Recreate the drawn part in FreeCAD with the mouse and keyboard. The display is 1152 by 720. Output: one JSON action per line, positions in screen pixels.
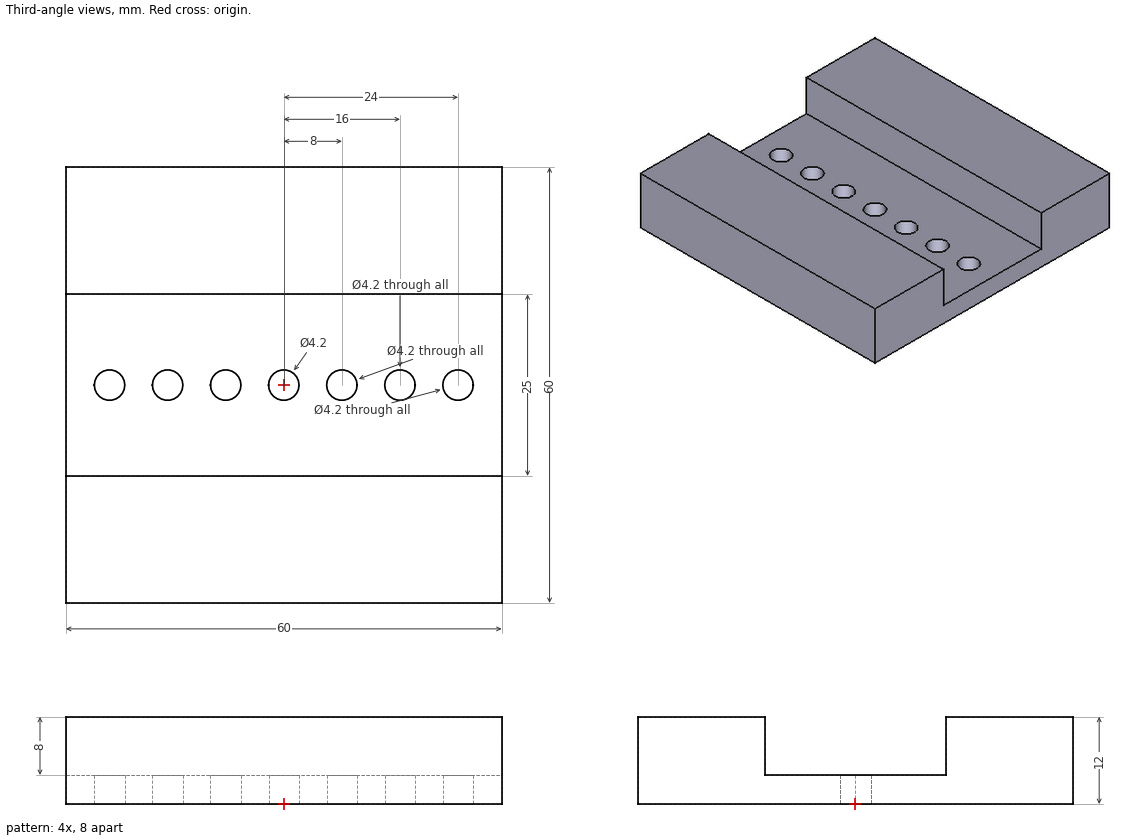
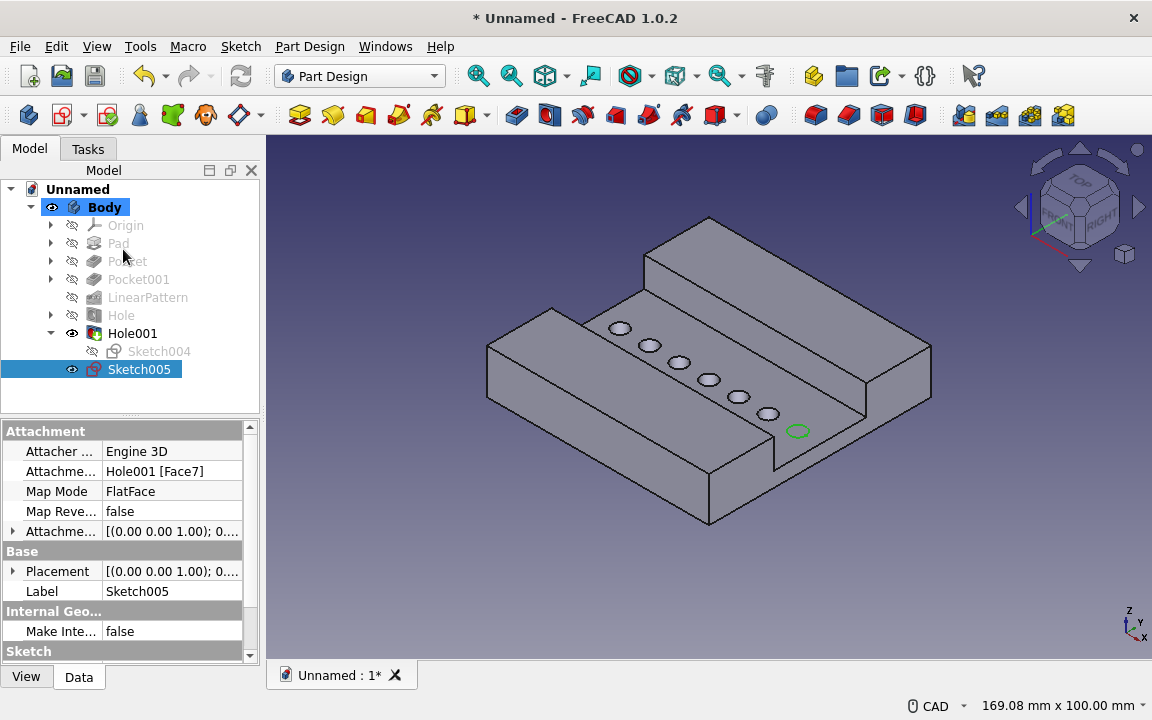
{"action": "left_click", "coordinate": [550, 116]}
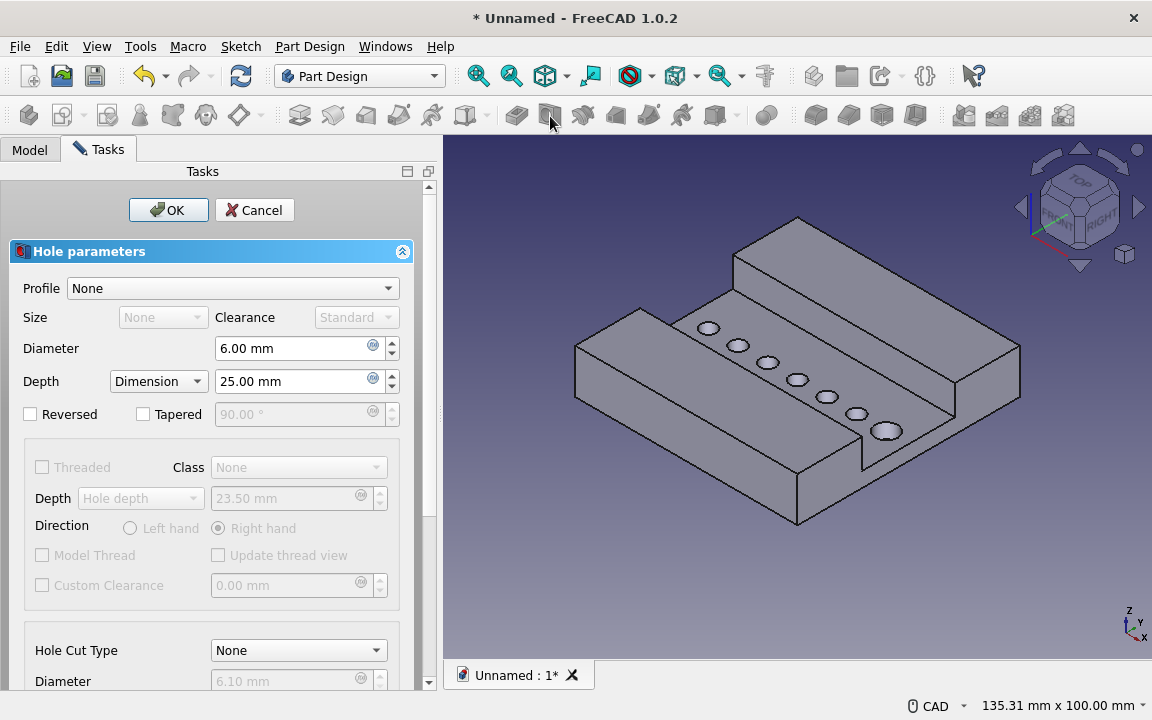
{"action": "triple_click", "coordinate": [300, 348]}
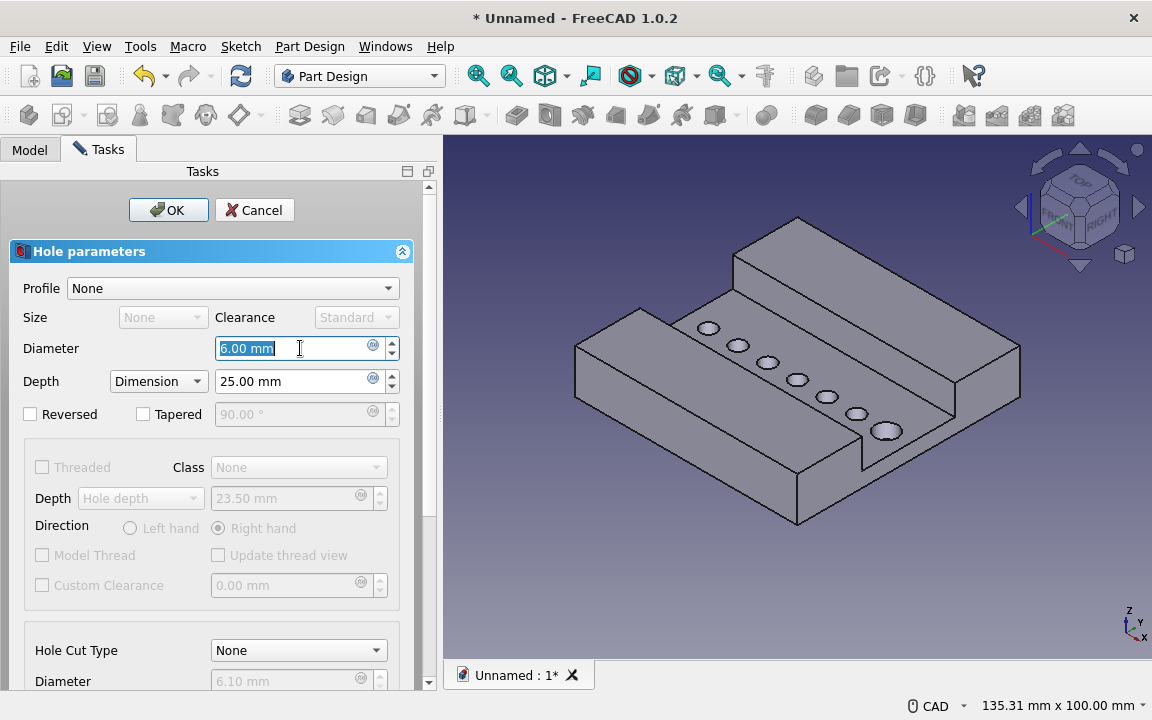
{"action": "type", "text": "4.2"}
{"action": "key", "text": "Tab"}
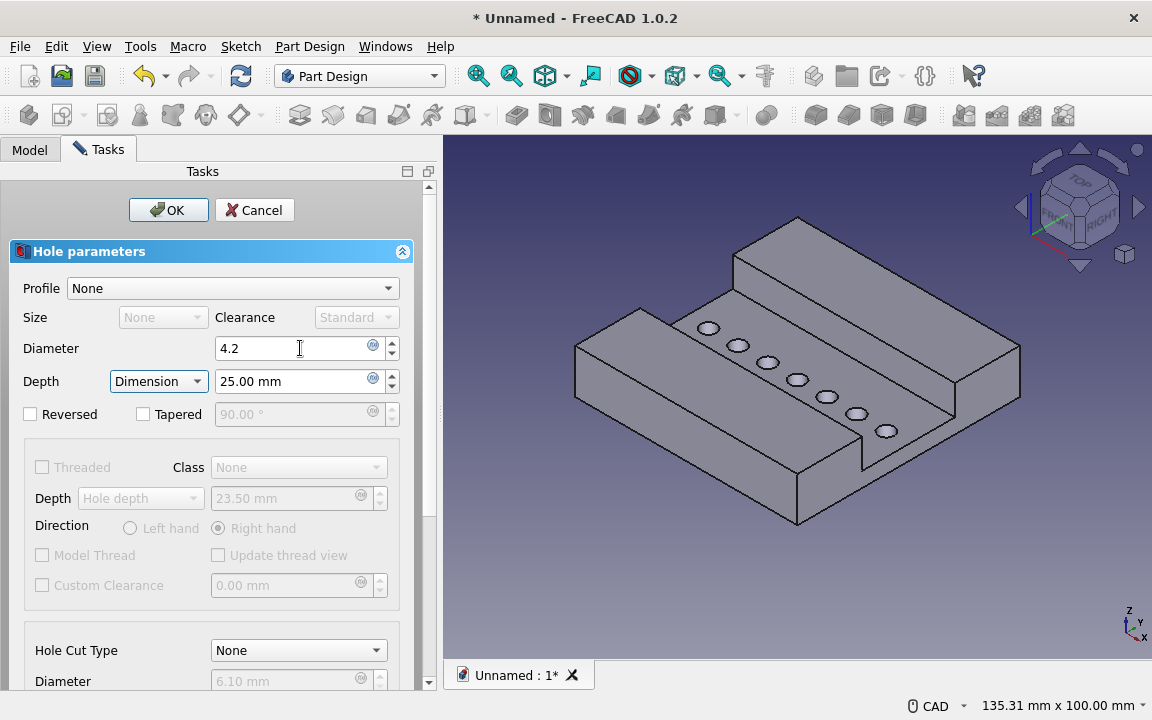
{"action": "left_click", "coordinate": [160, 382]}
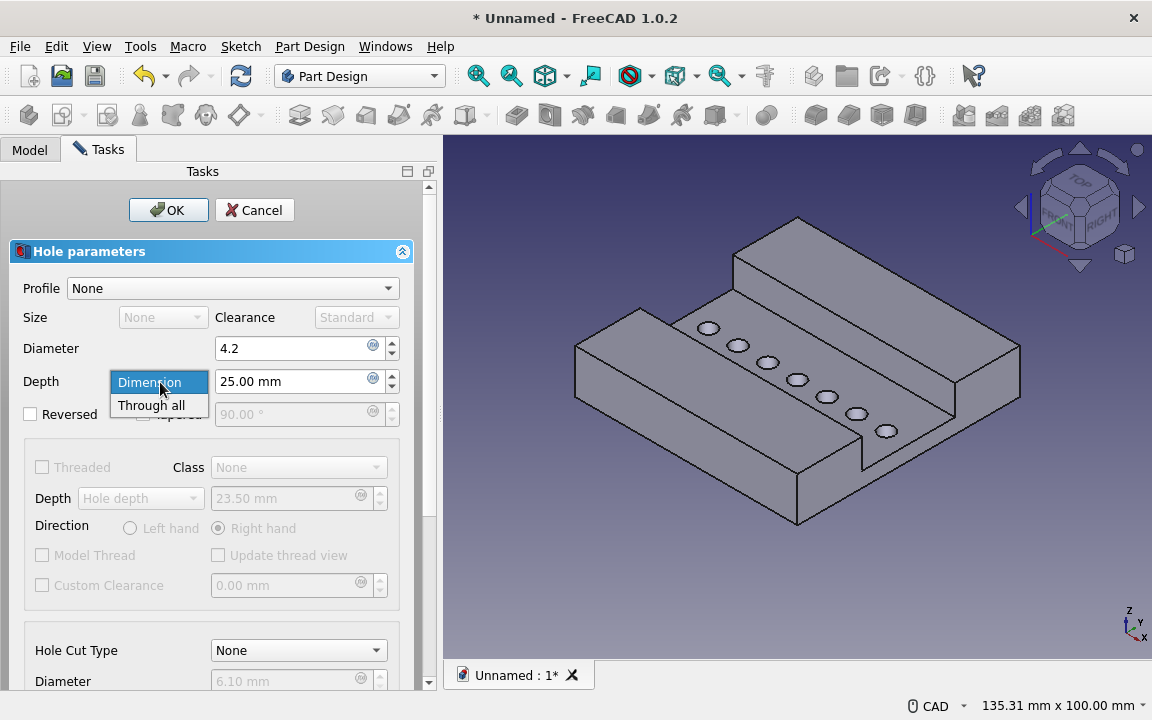
{"action": "left_click", "coordinate": [158, 406]}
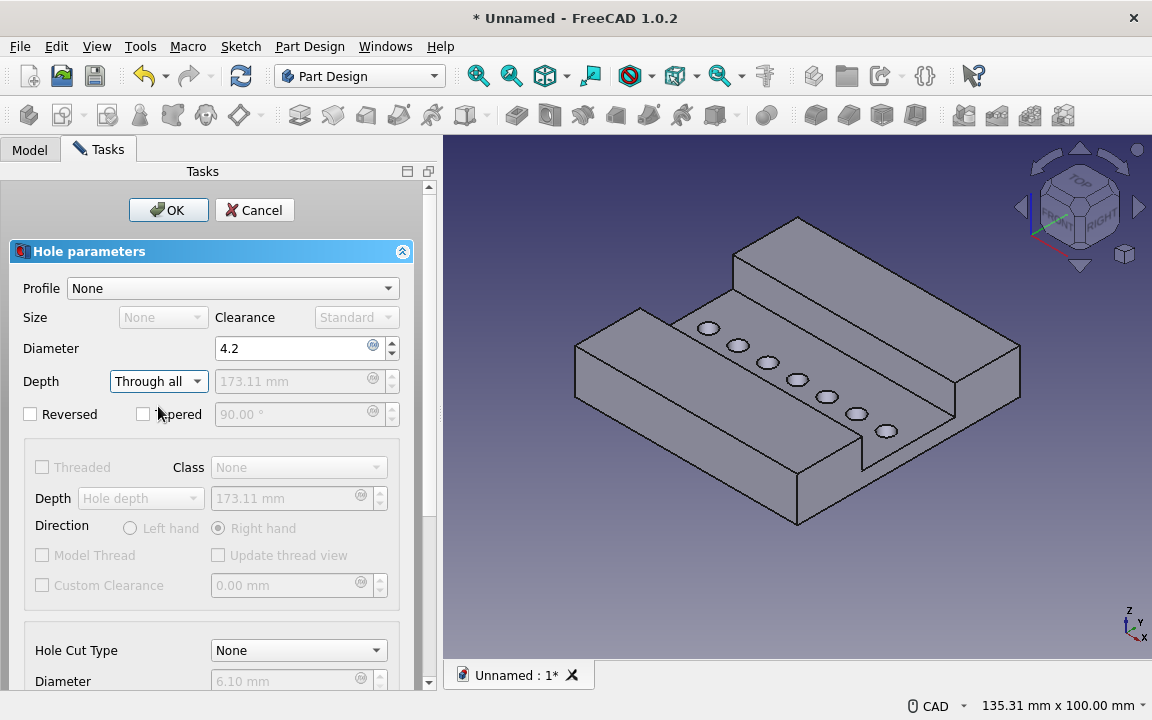
{"action": "left_click", "coordinate": [169, 210]}